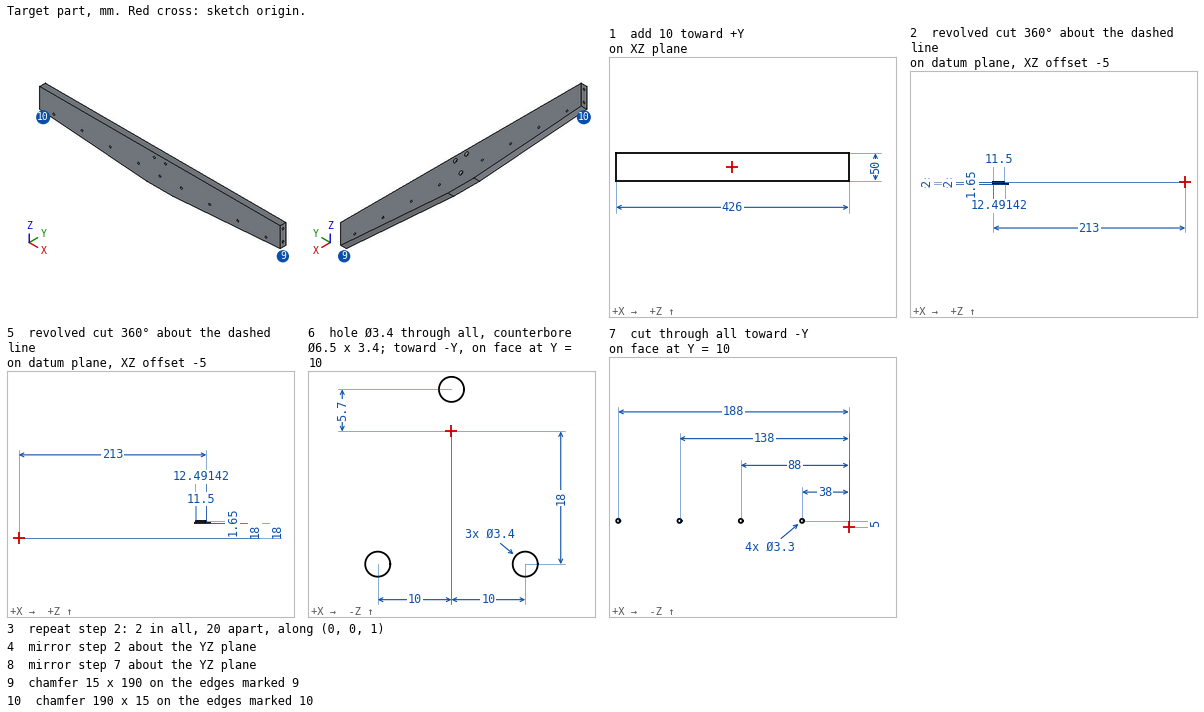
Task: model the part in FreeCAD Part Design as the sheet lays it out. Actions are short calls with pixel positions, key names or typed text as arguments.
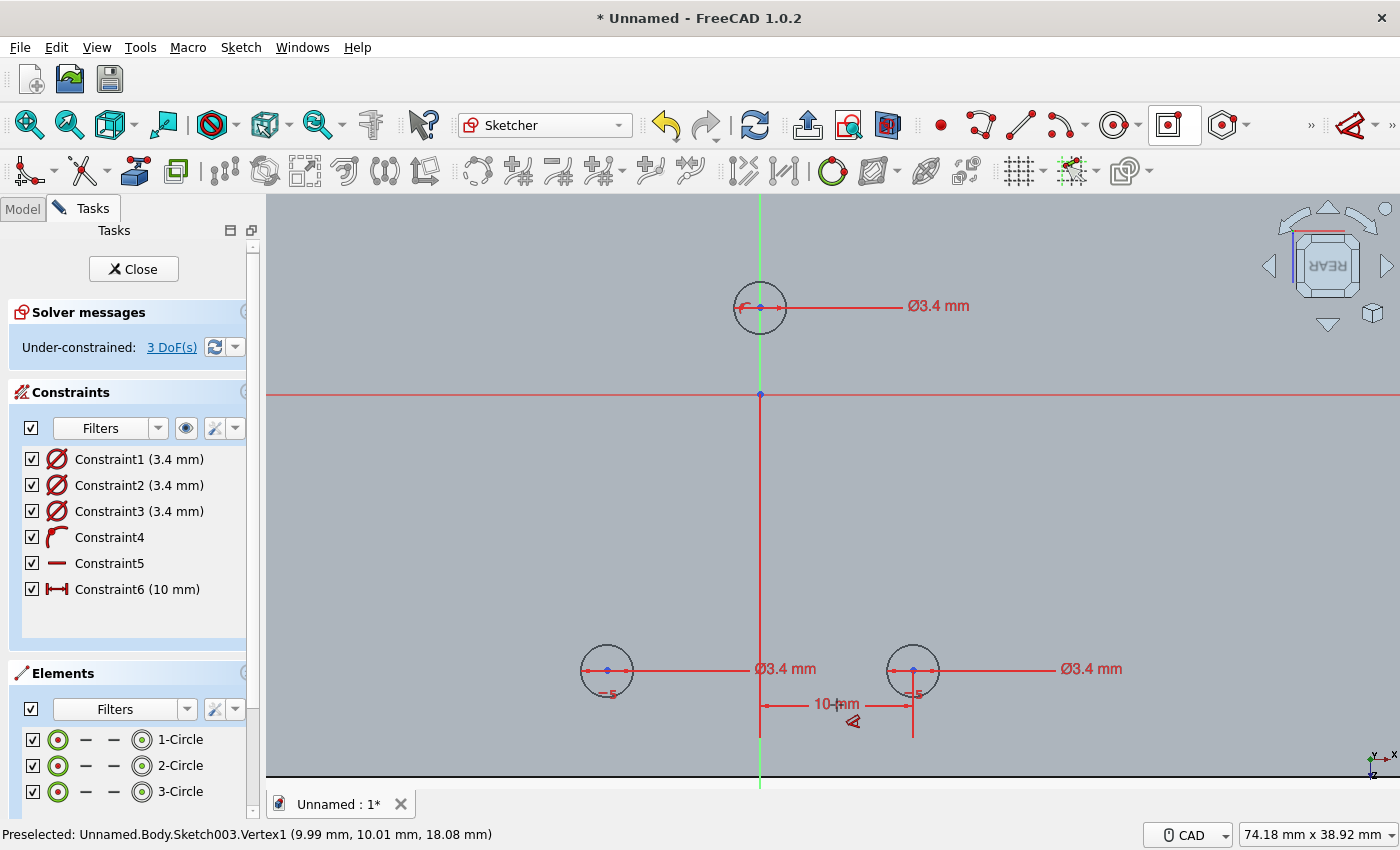
click(913, 671)
click(947, 533)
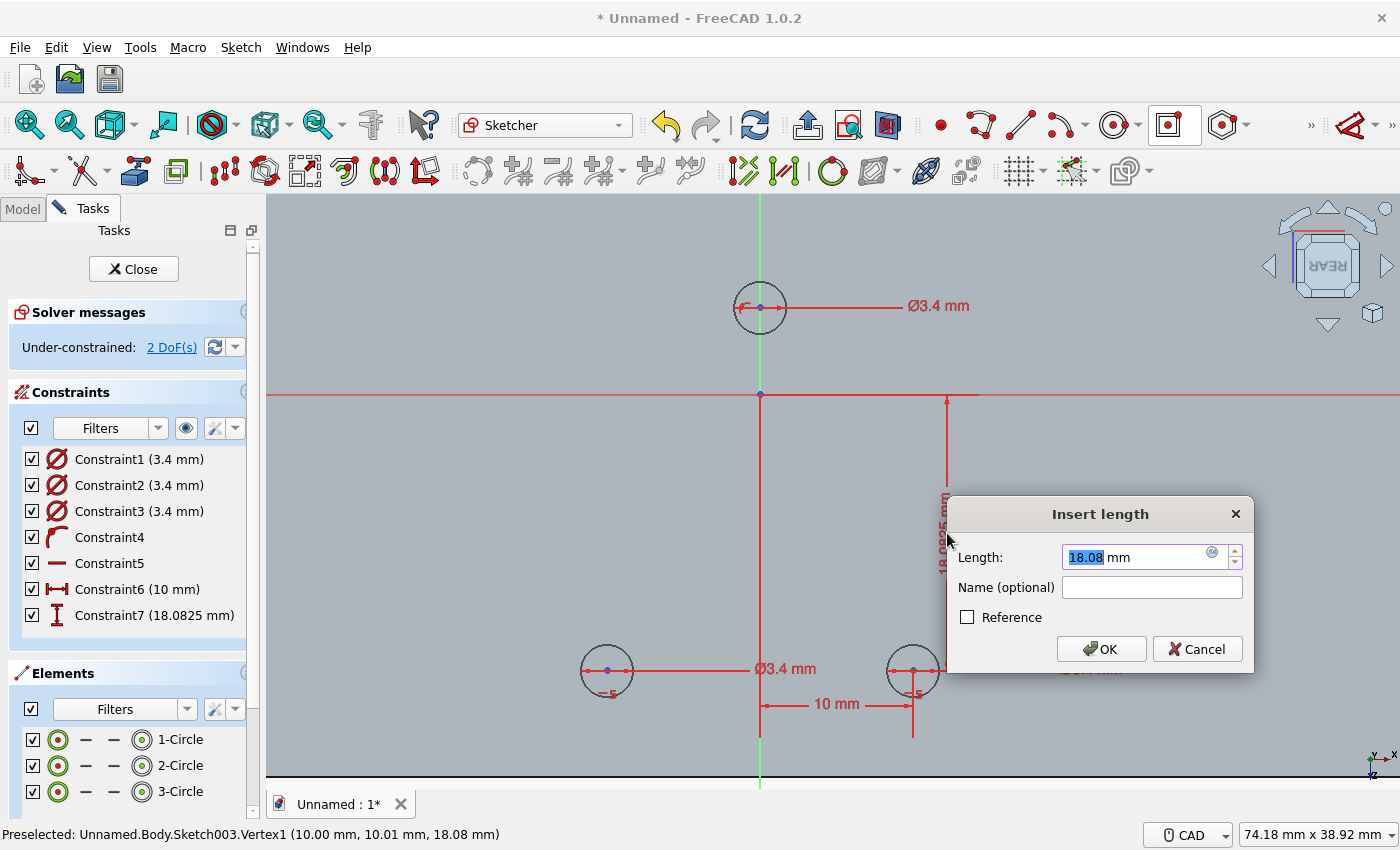
text(18)
key(Return)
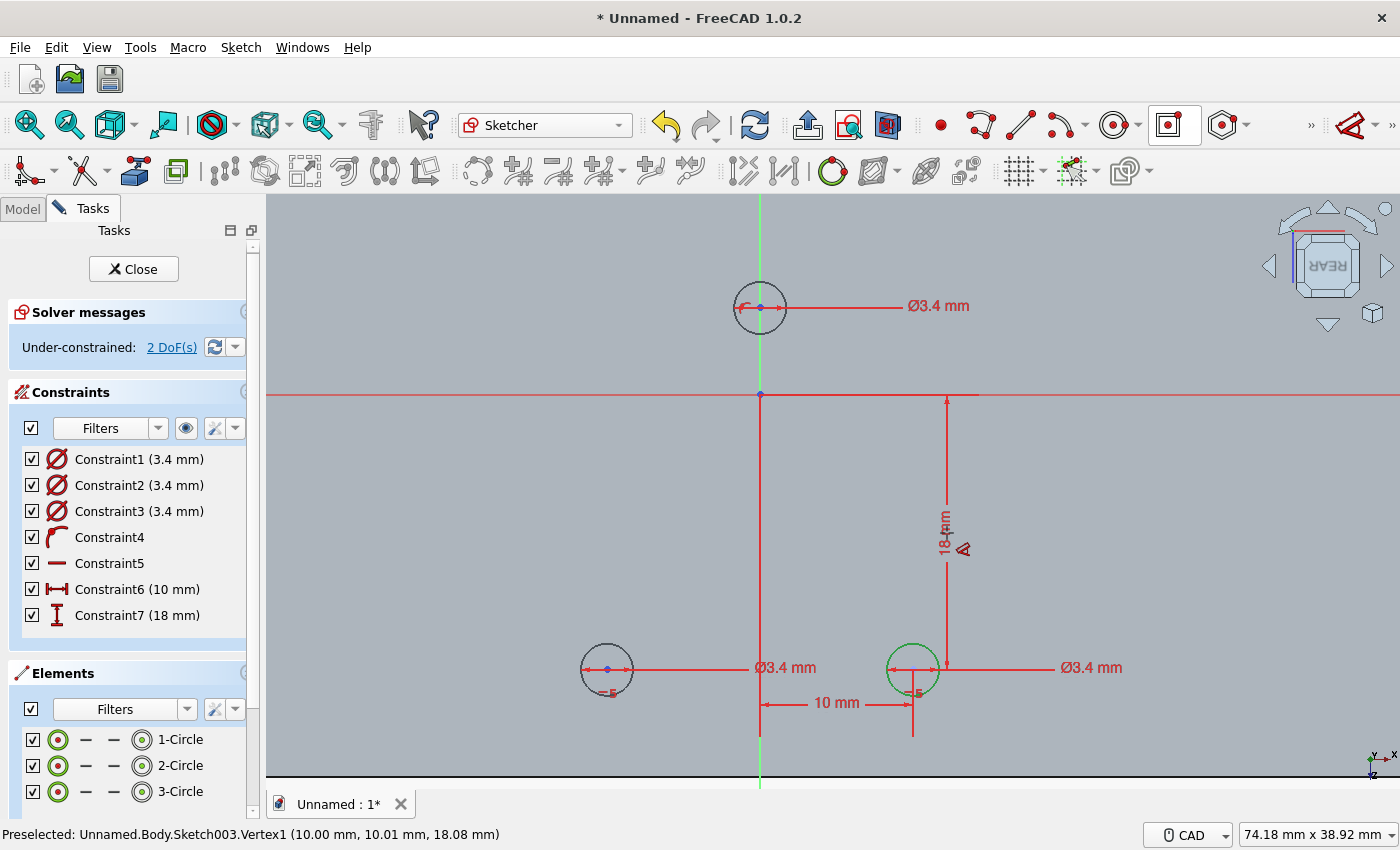
click(607, 670)
click(684, 704)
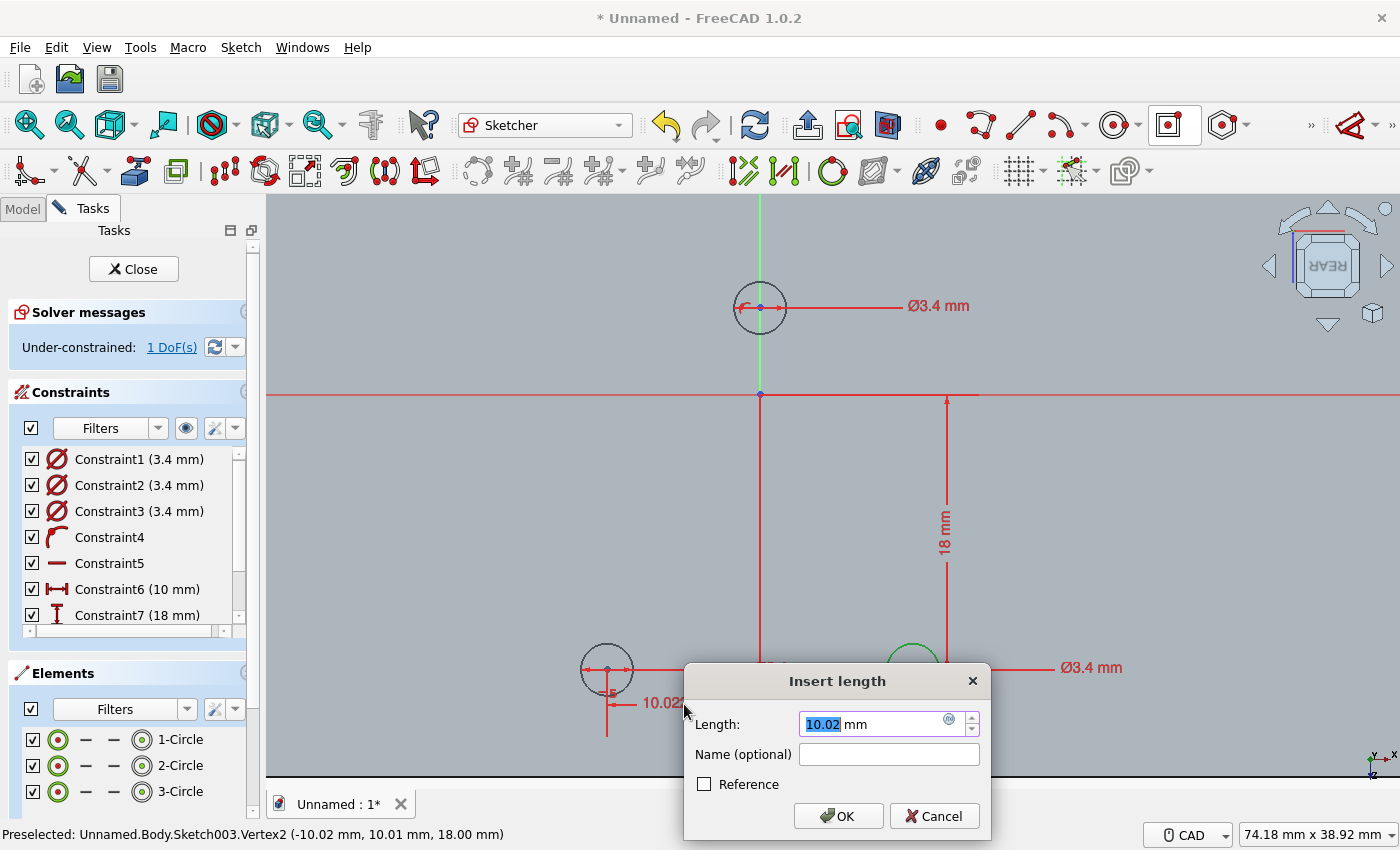
text(10)
key(Return)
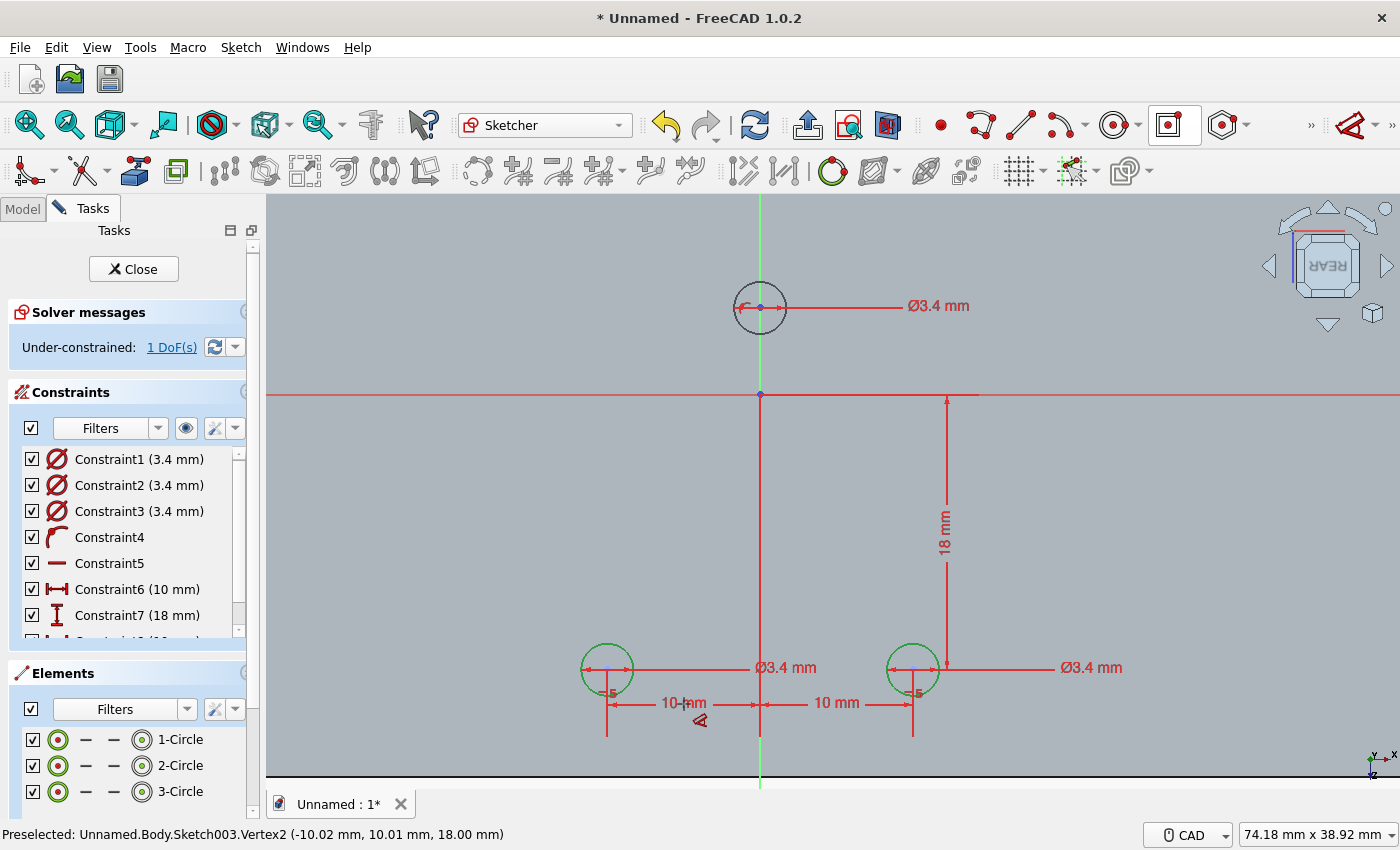
click(760, 308)
click(794, 351)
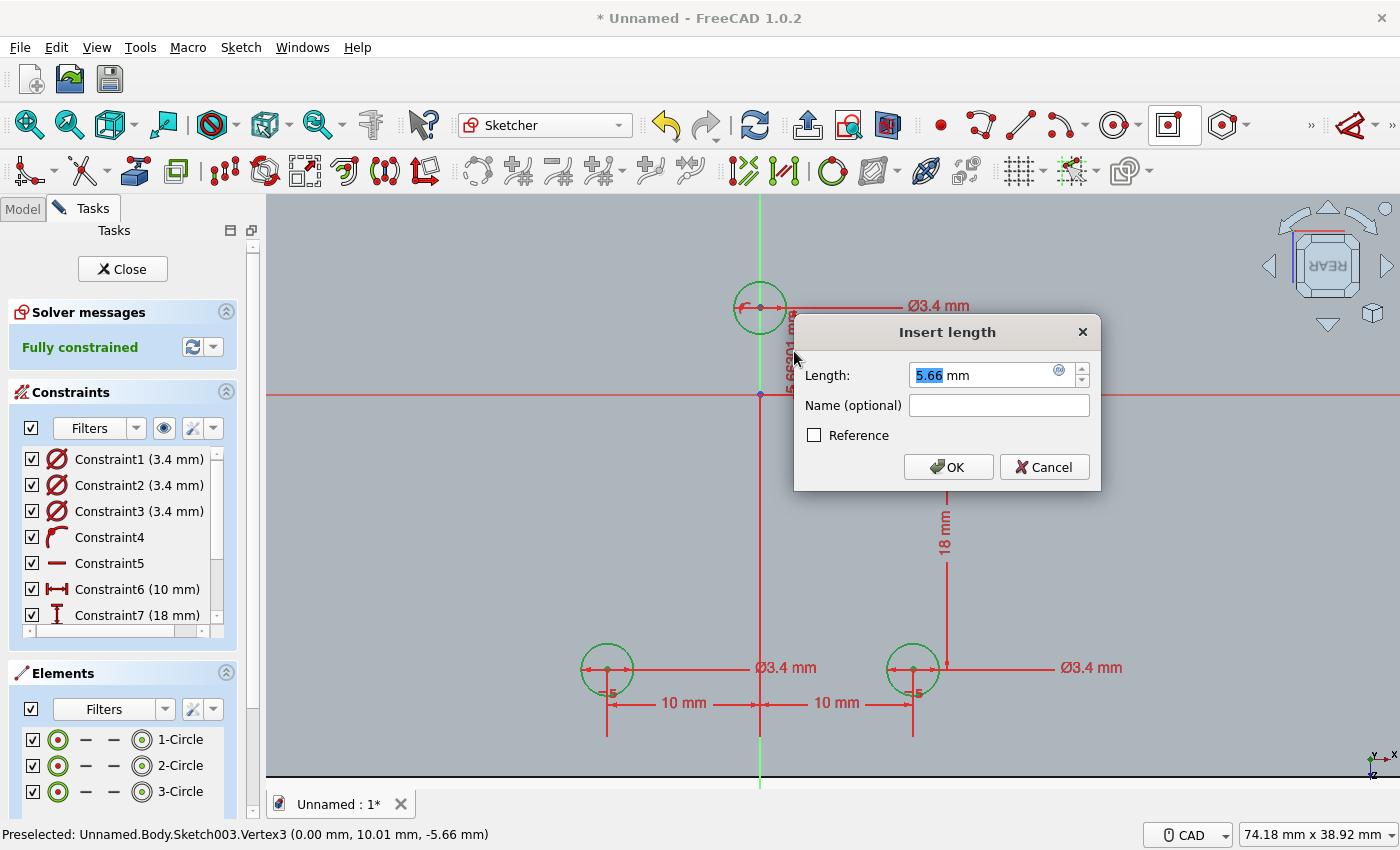
text(5.7)
key(Return)
key(Escape)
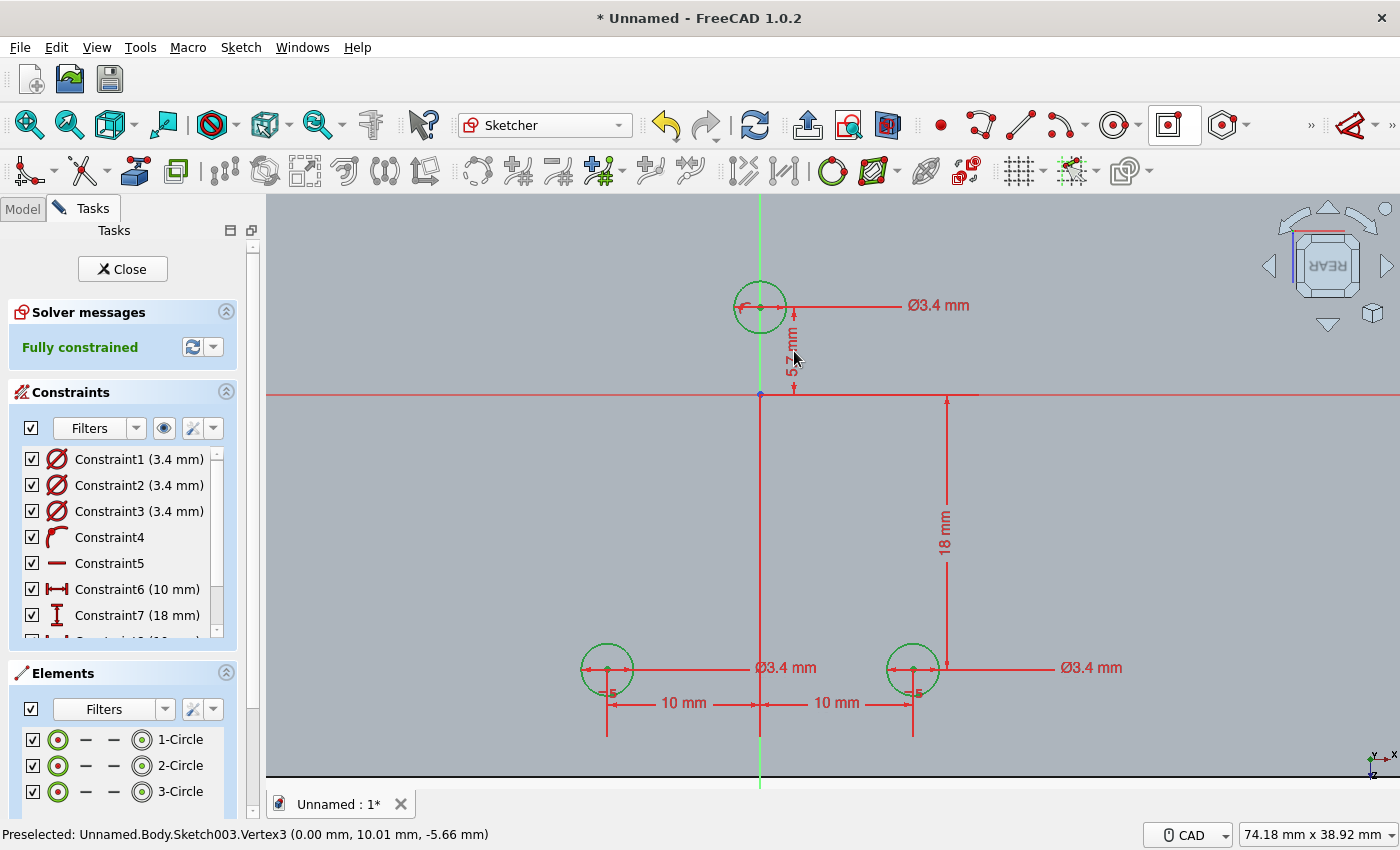
click(123, 269)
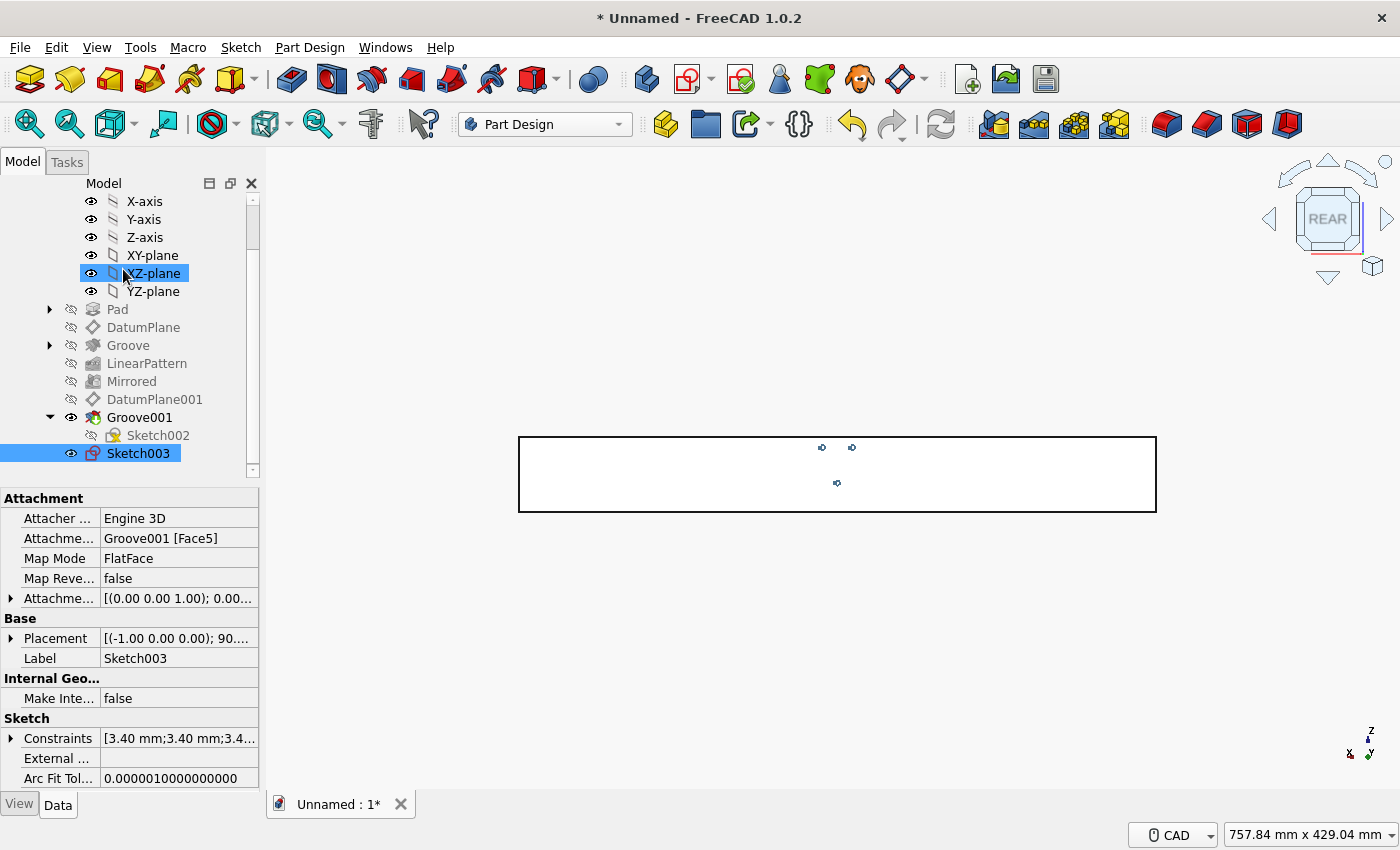
click(332, 80)